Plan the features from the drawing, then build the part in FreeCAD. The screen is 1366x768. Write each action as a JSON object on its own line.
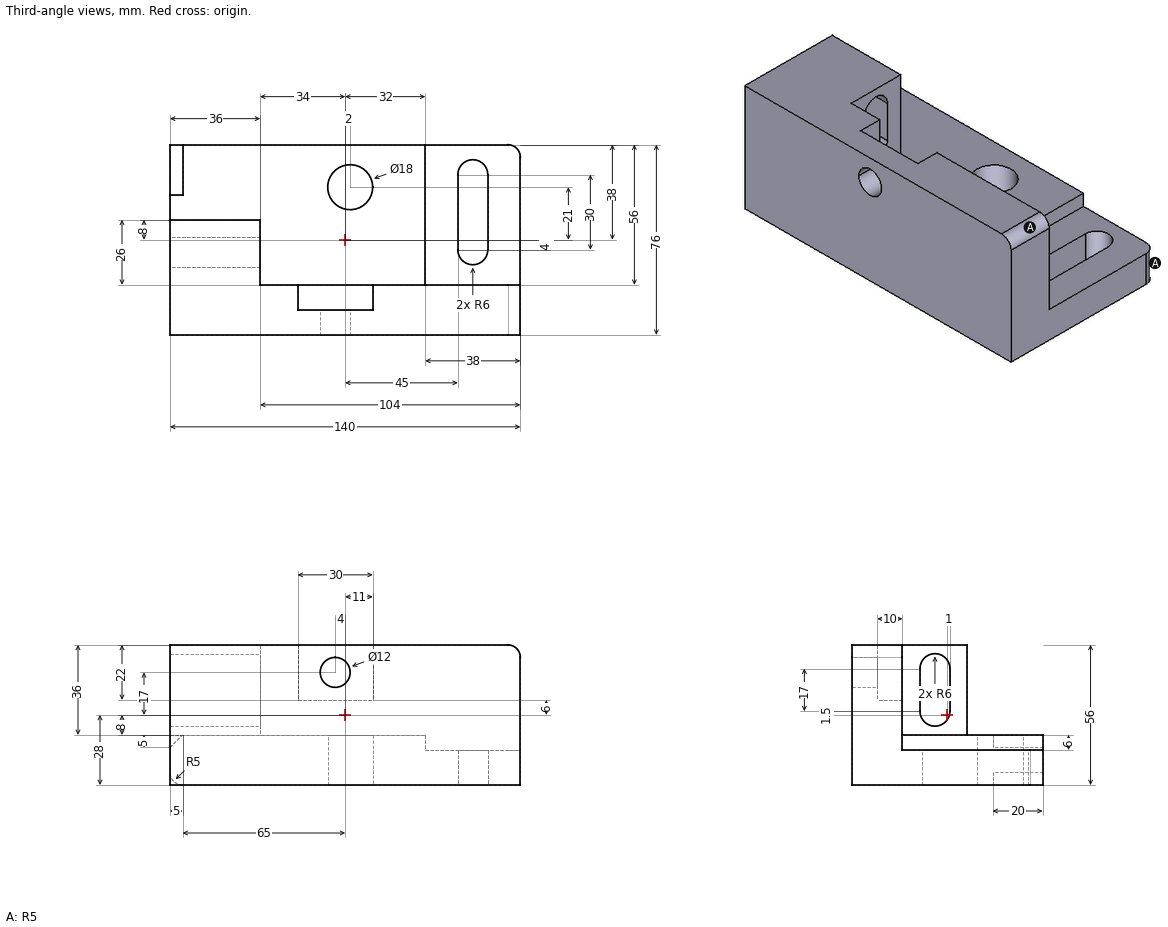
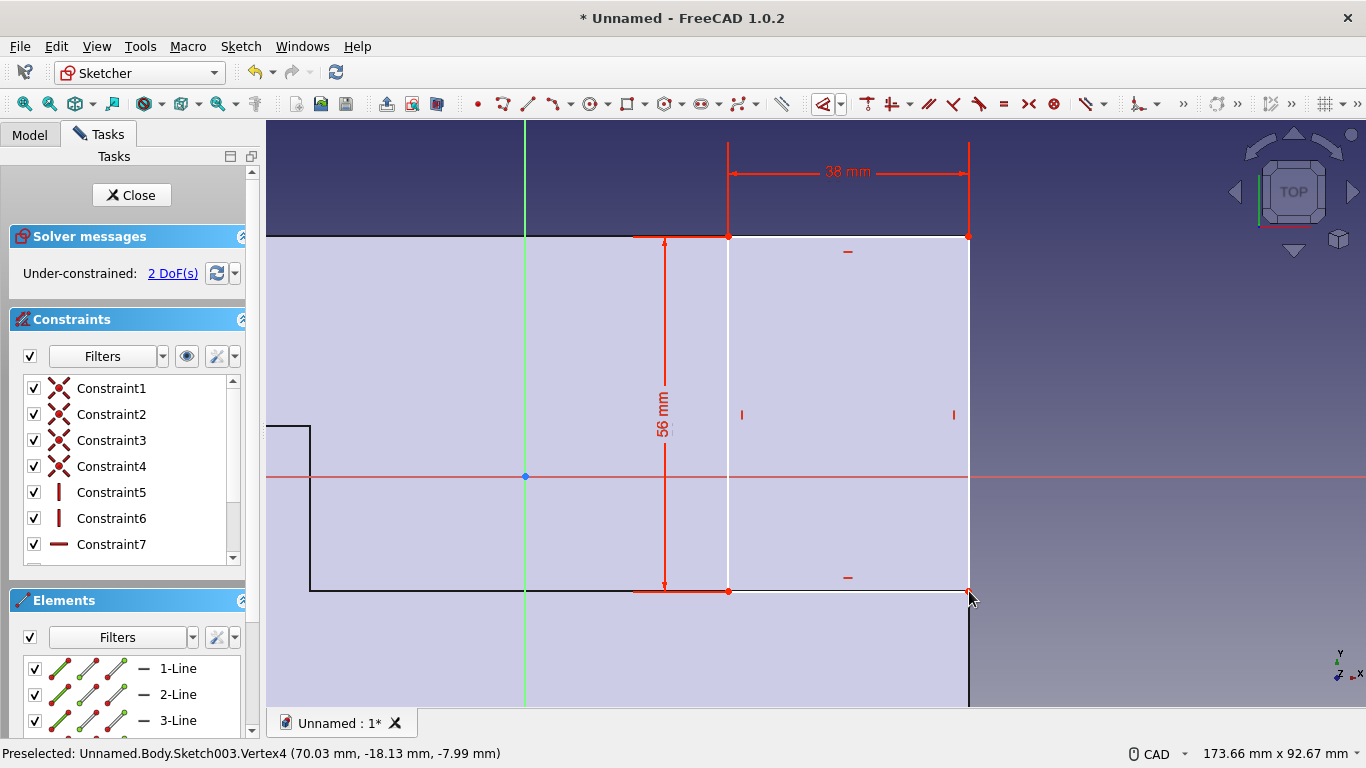
{"action": "left_click", "coordinate": [728, 237]}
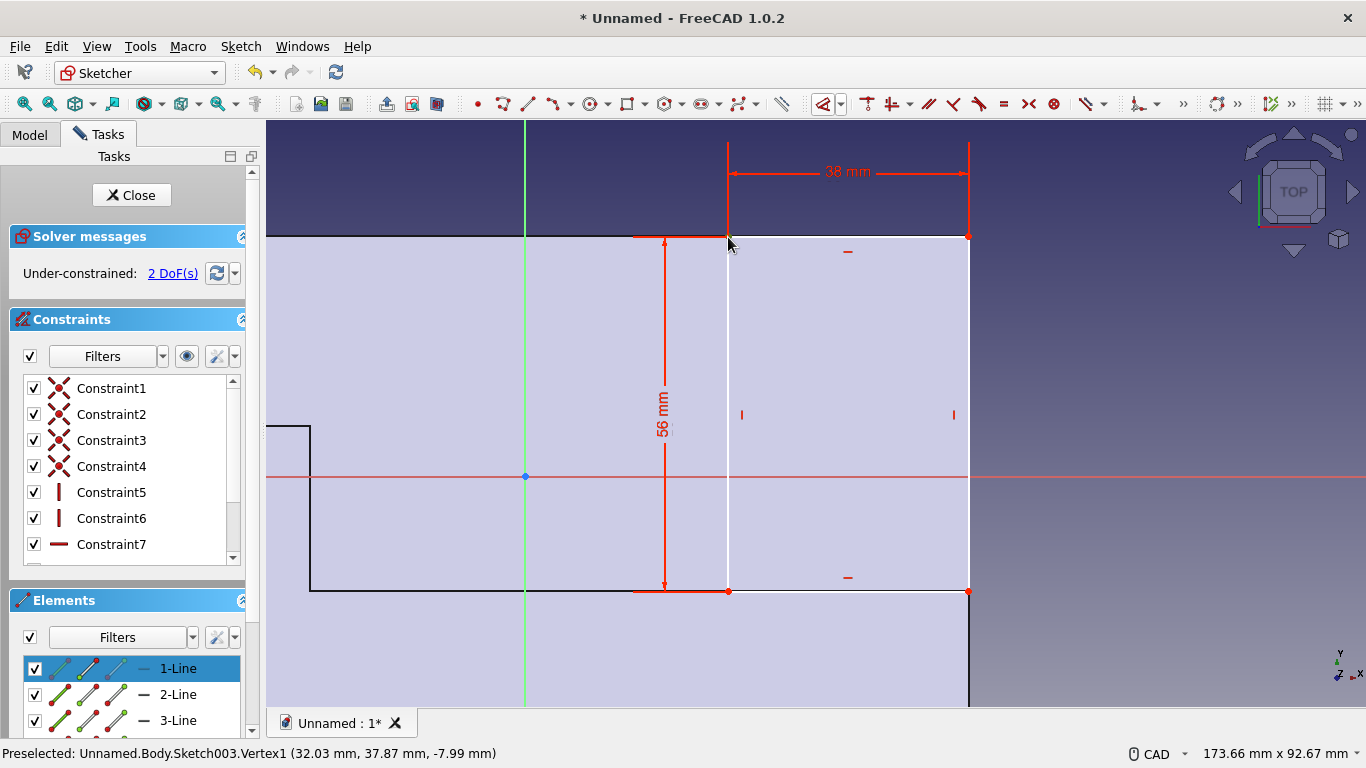
{"action": "left_click", "coordinate": [840, 104]}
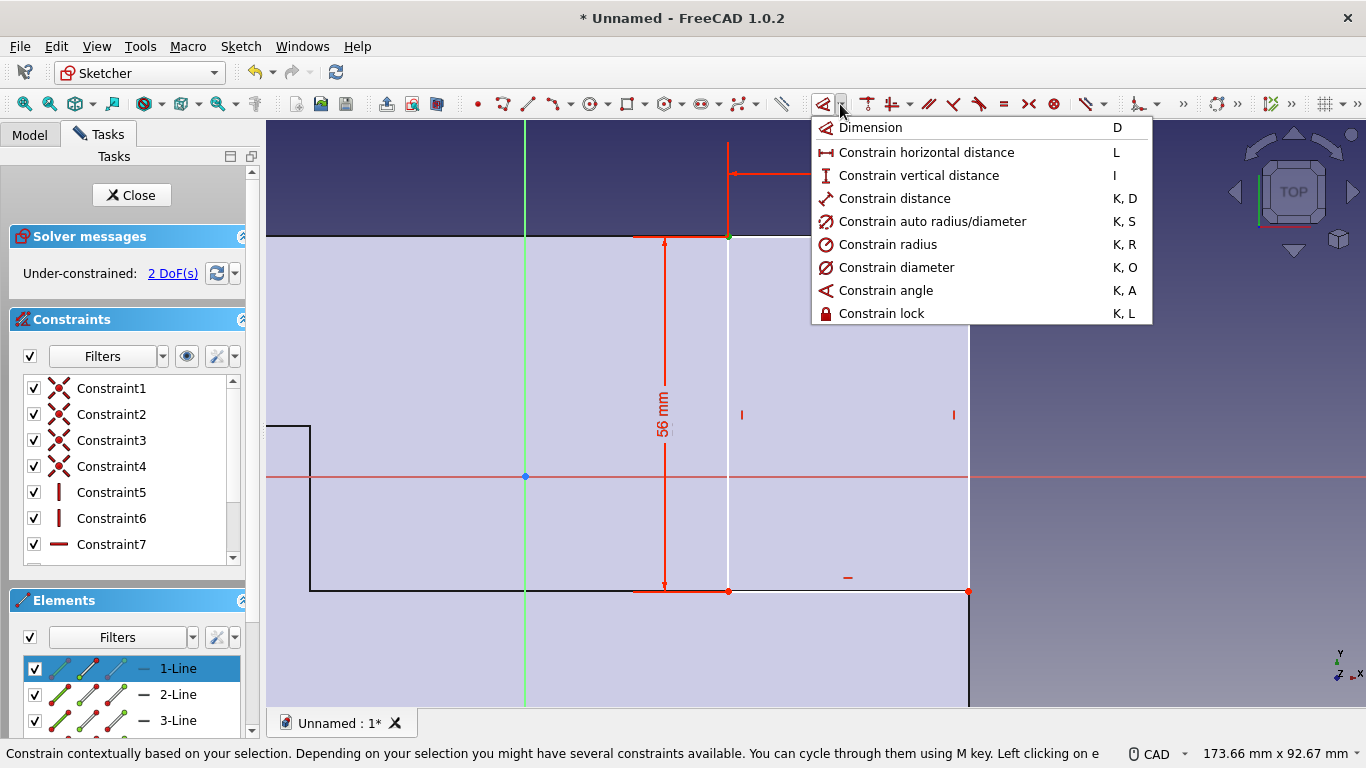
{"action": "left_click", "coordinate": [982, 152]}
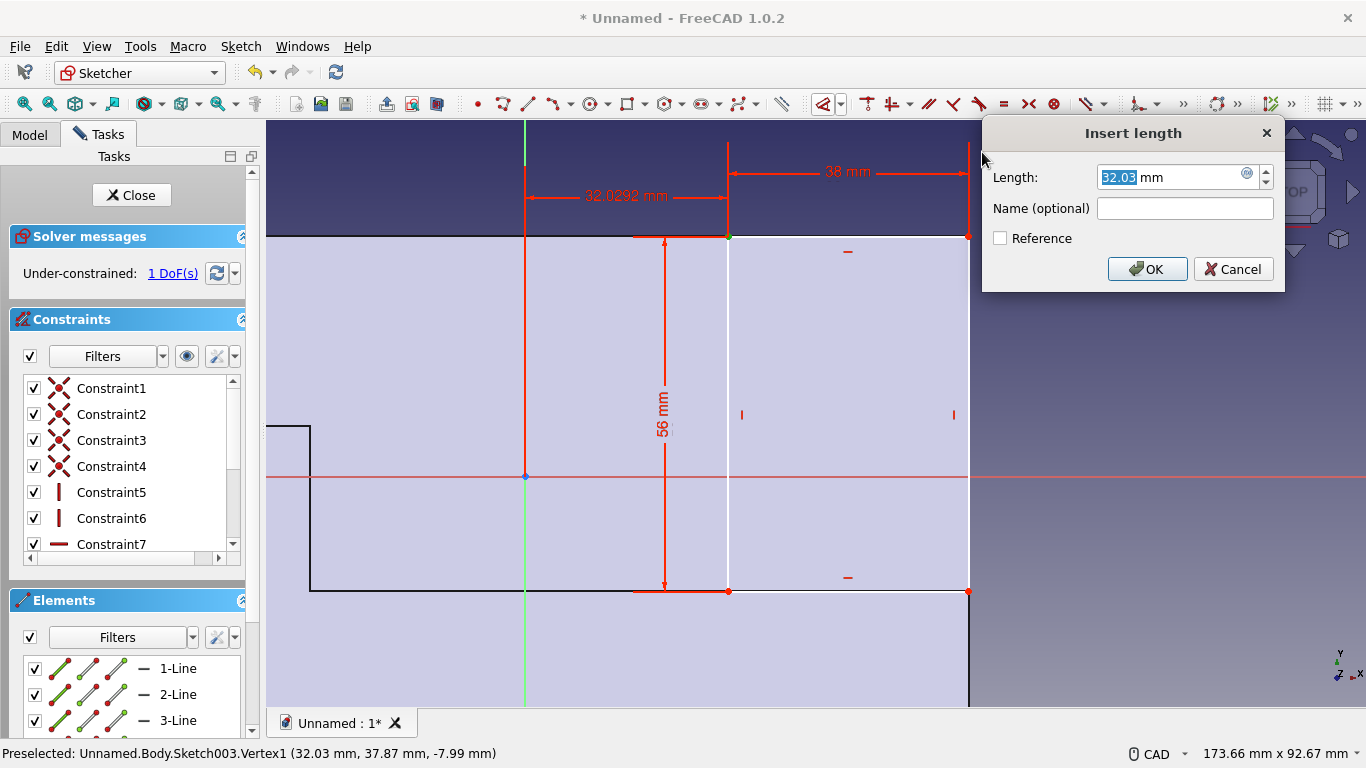
{"action": "type", "text": "32"}
{"action": "key", "text": "Return"}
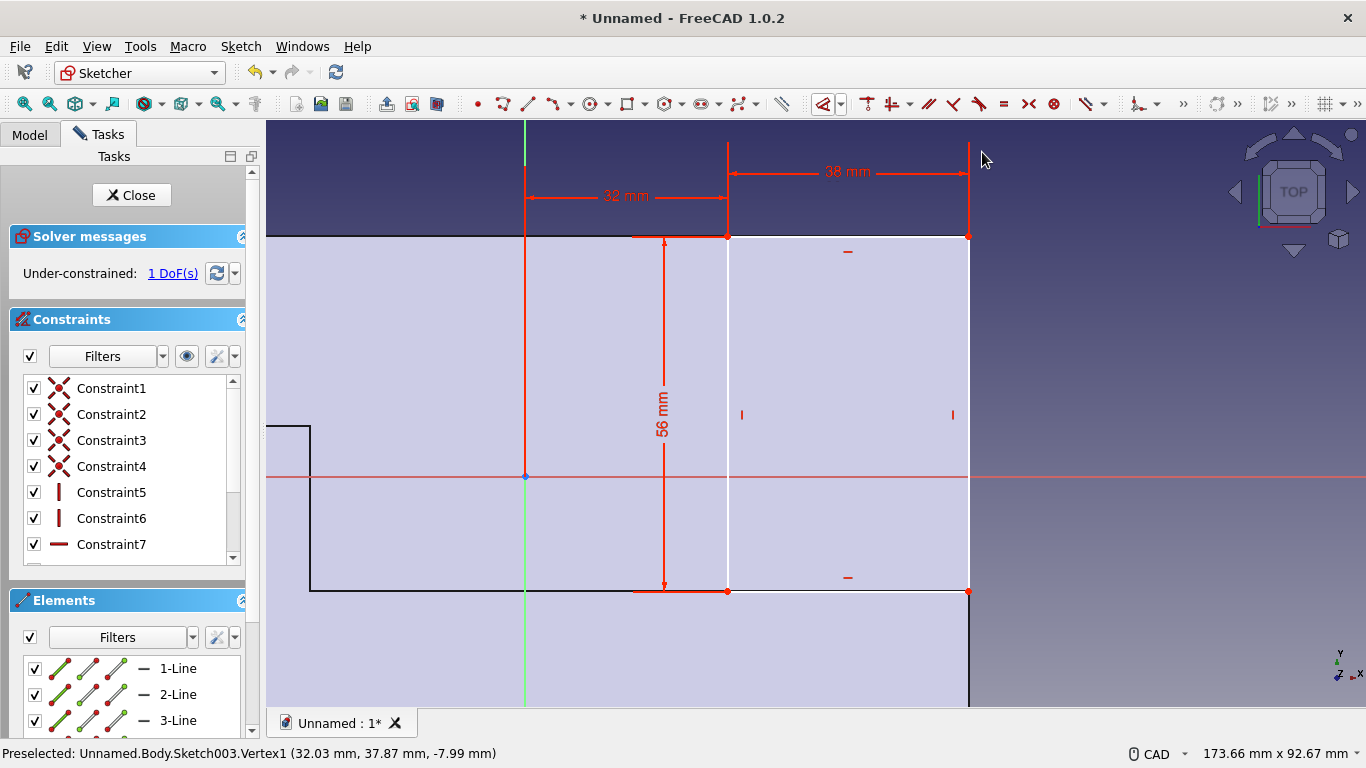
{"action": "left_click", "coordinate": [728, 237]}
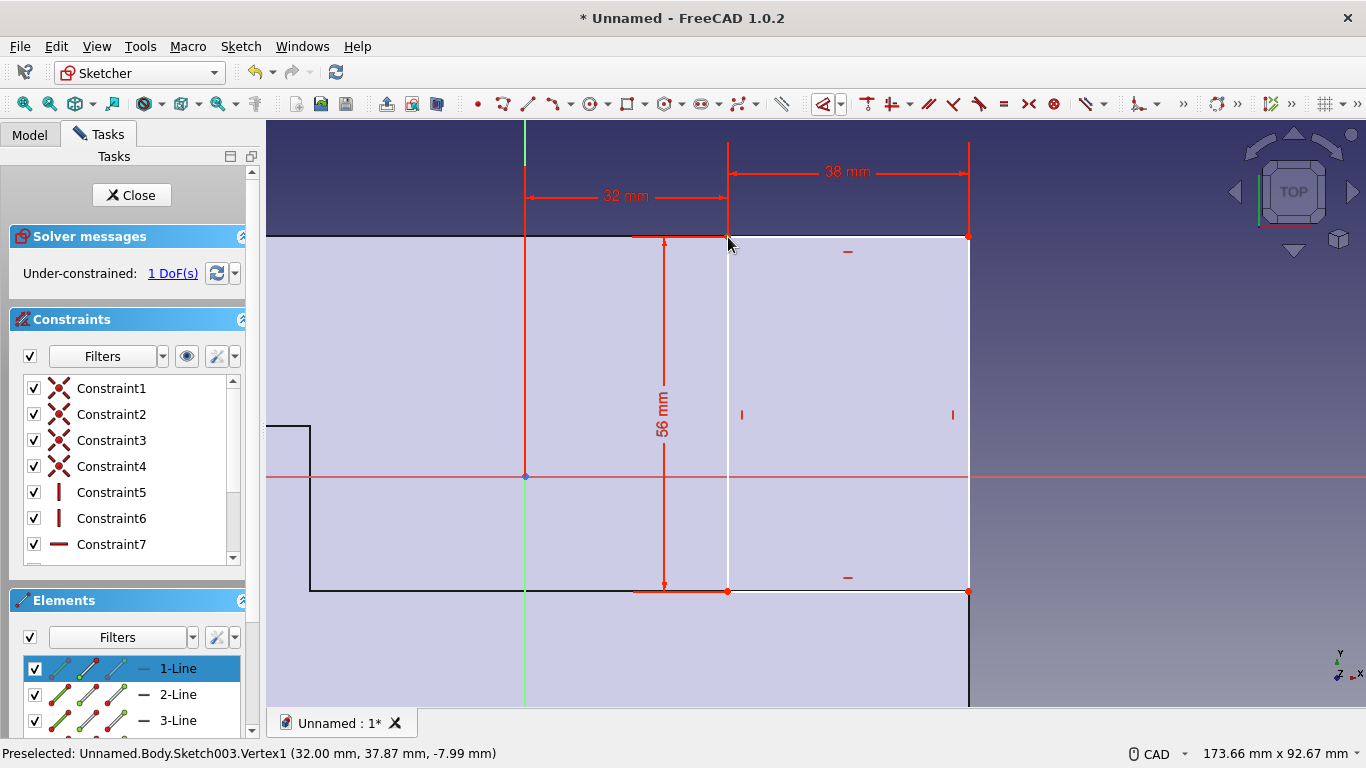
{"action": "key", "text": "i"}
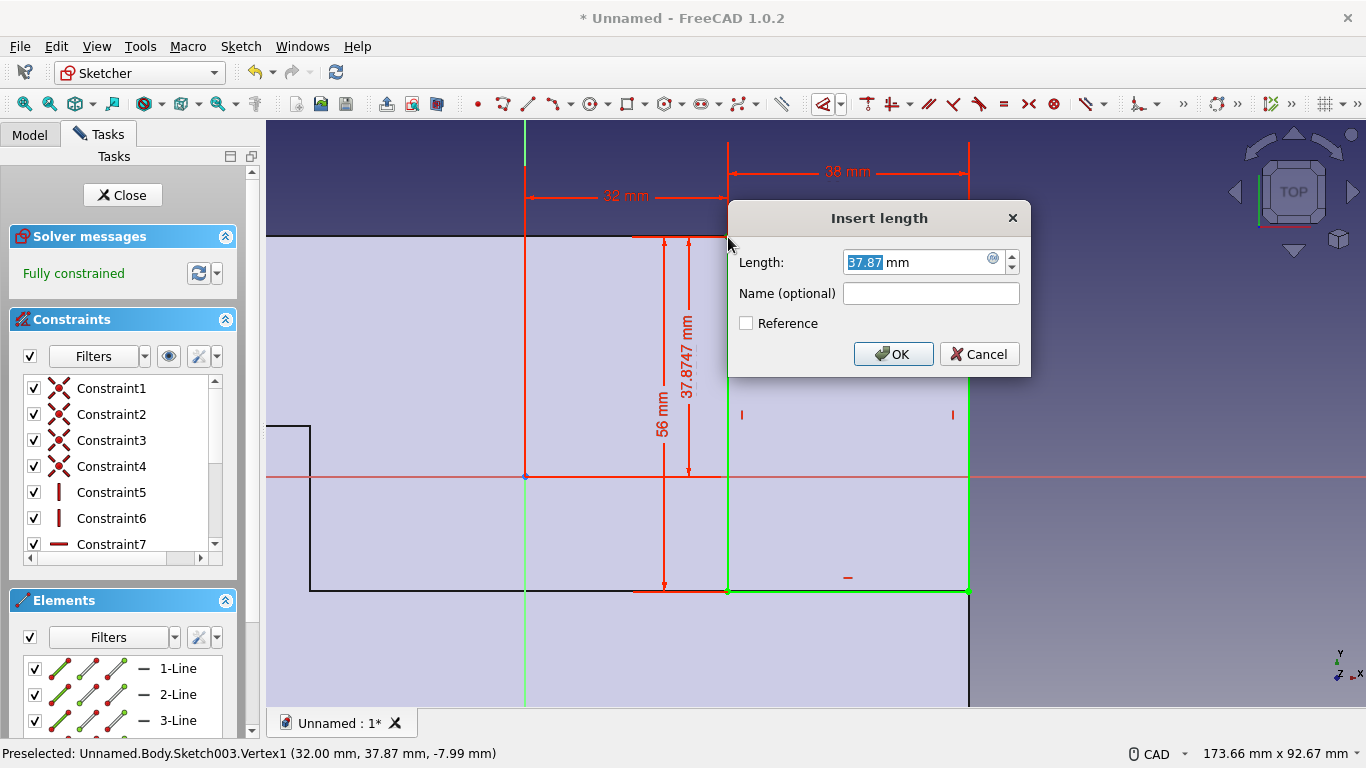
{"action": "type", "text": "38"}
{"action": "key", "text": "Return"}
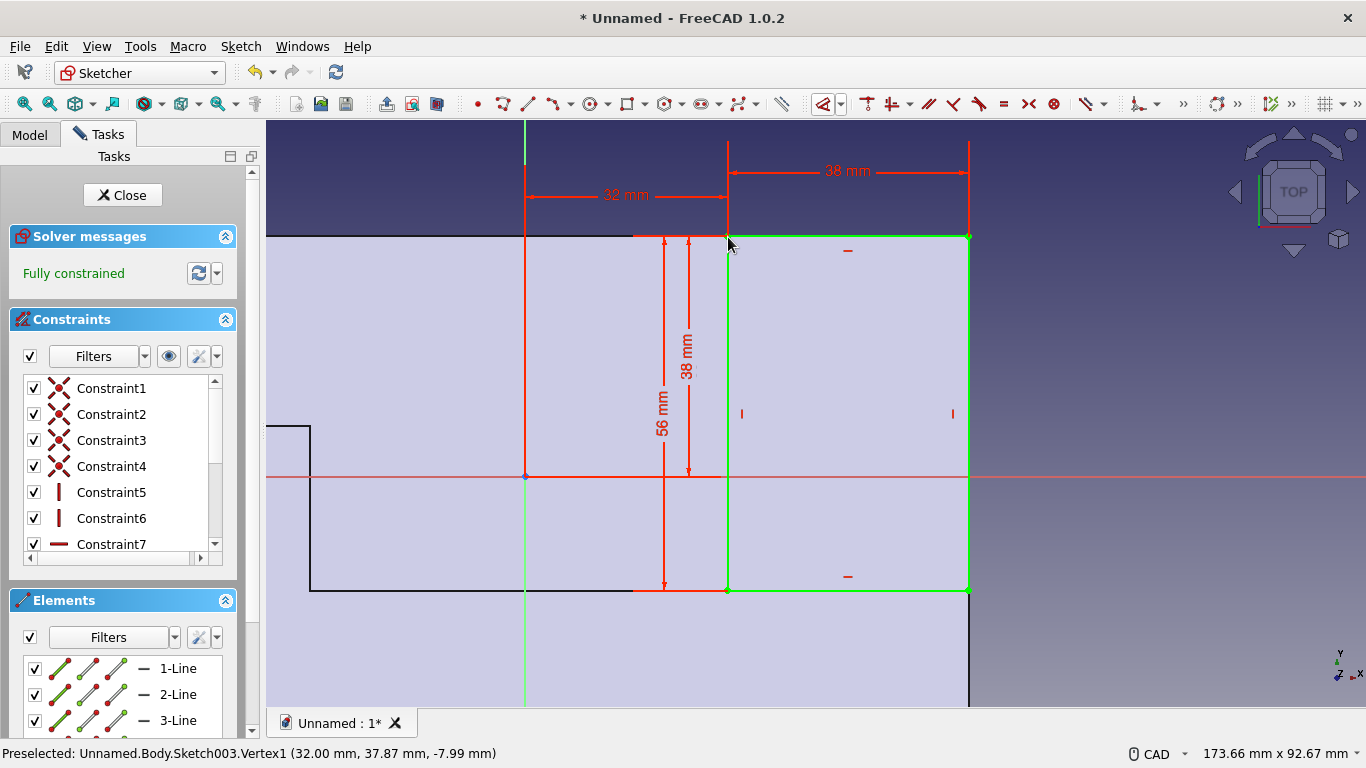
{"action": "left_click", "coordinate": [123, 195]}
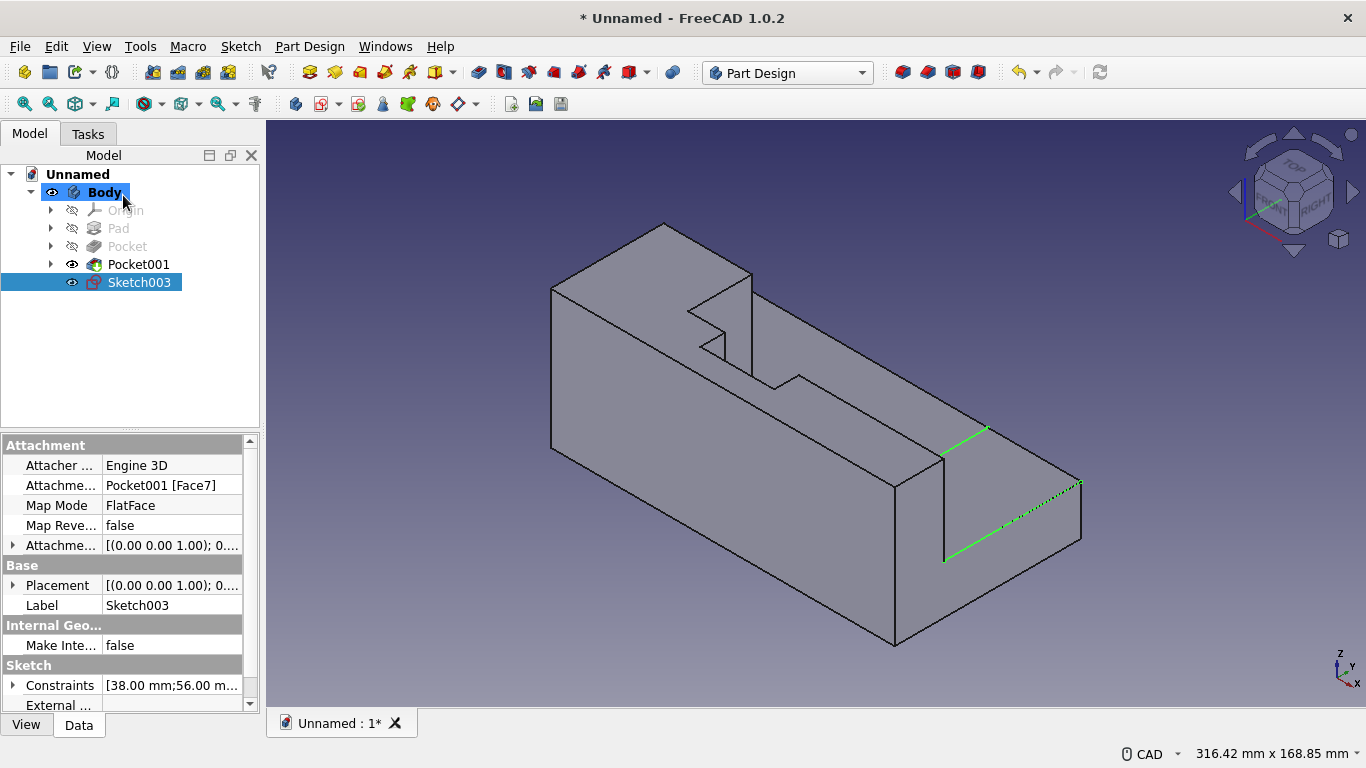
{"action": "left_click", "coordinate": [479, 72]}